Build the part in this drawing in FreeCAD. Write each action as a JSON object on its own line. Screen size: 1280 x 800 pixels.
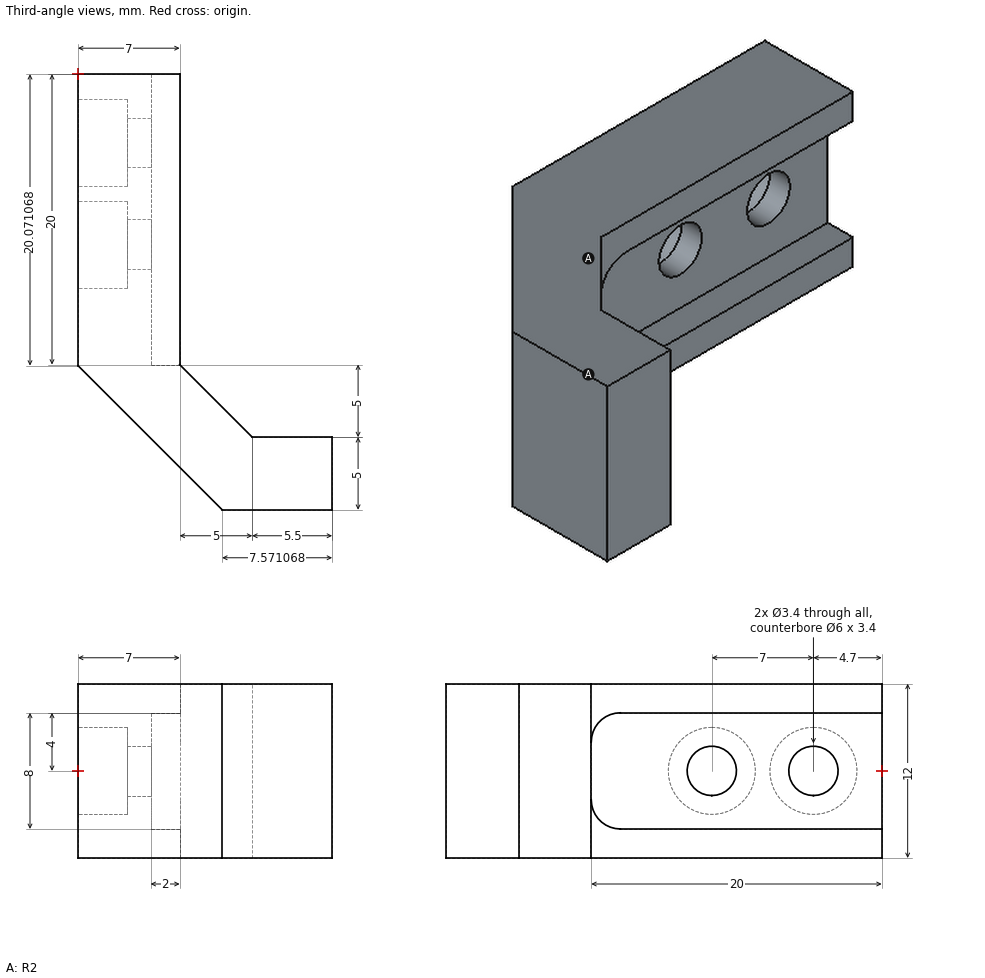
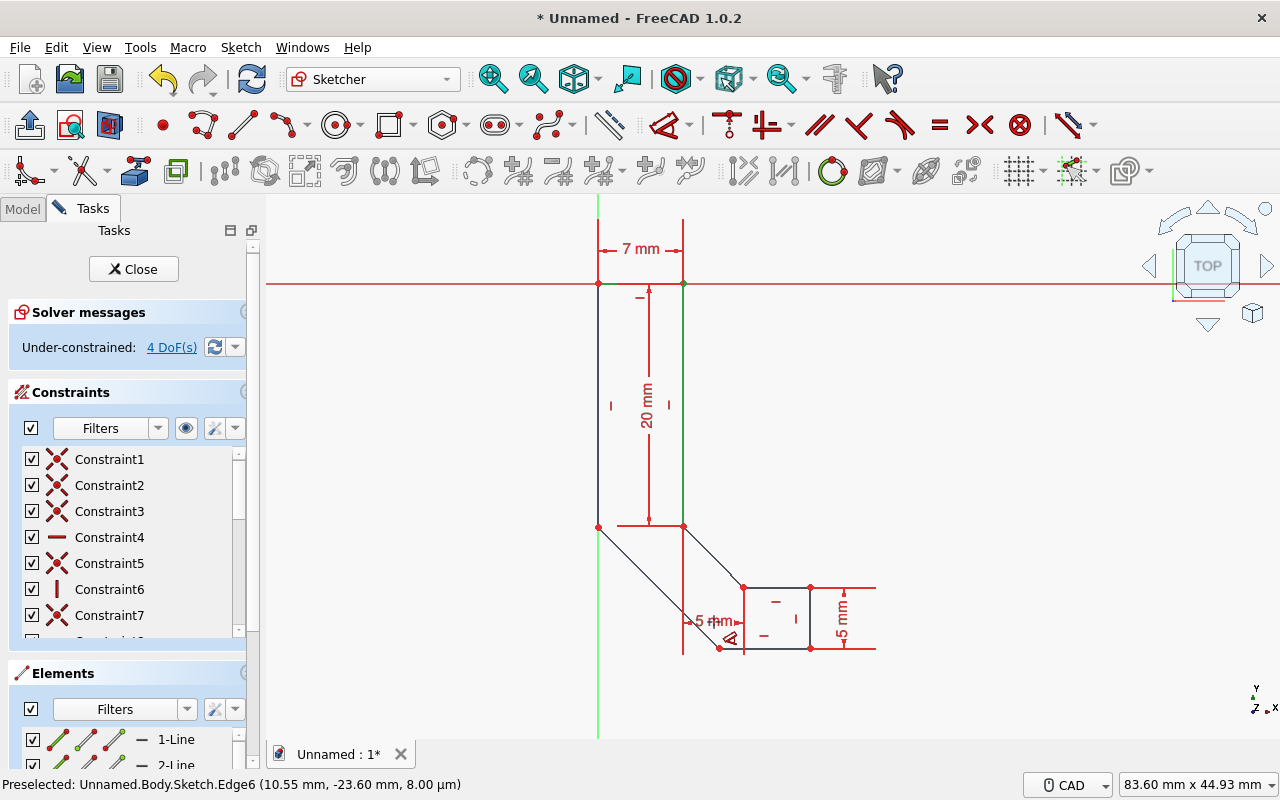
{"action": "left_click", "coordinate": [726, 569]}
{"action": "left_click", "coordinate": [778, 557]}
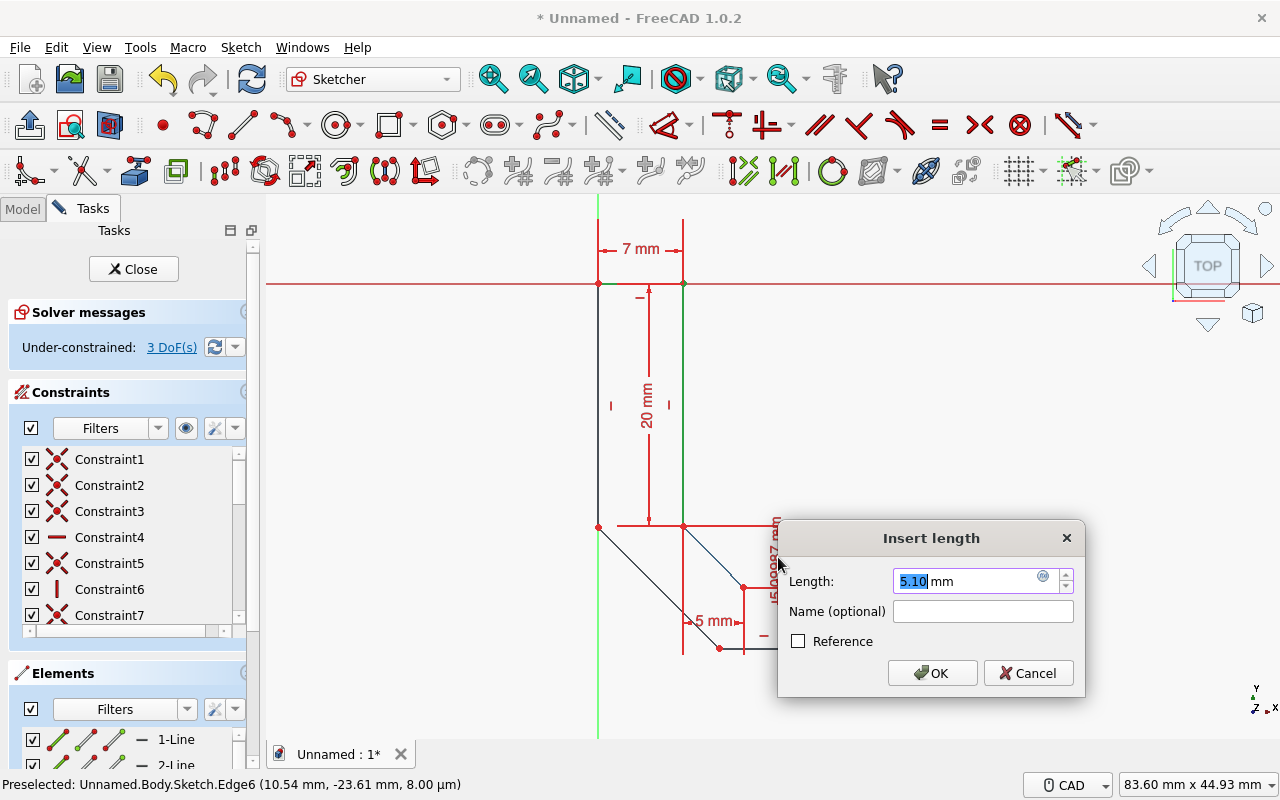
{"action": "type", "text": "5"}
{"action": "key", "text": "Return"}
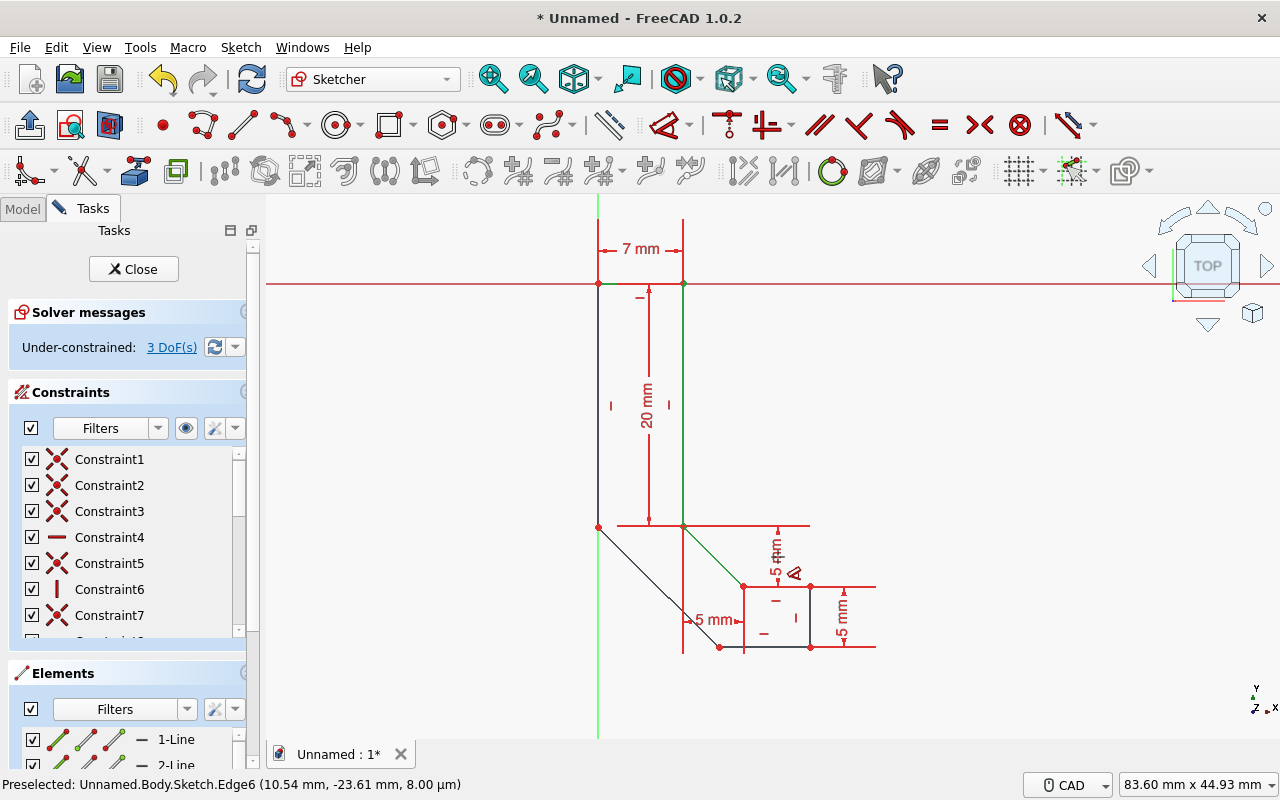
{"action": "left_click", "coordinate": [790, 587]}
{"action": "left_click", "coordinate": [777, 529]}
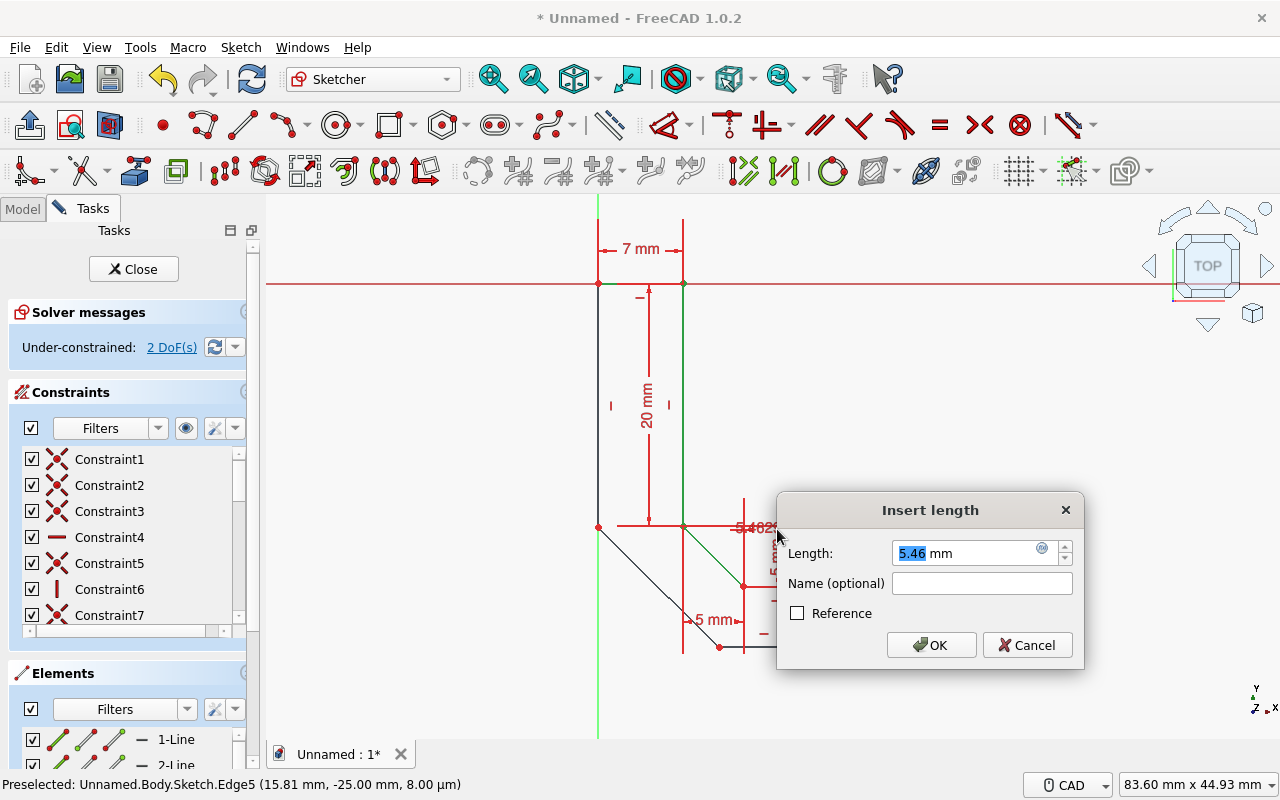
{"action": "type", "text": "5.5"}
{"action": "key", "text": "Return"}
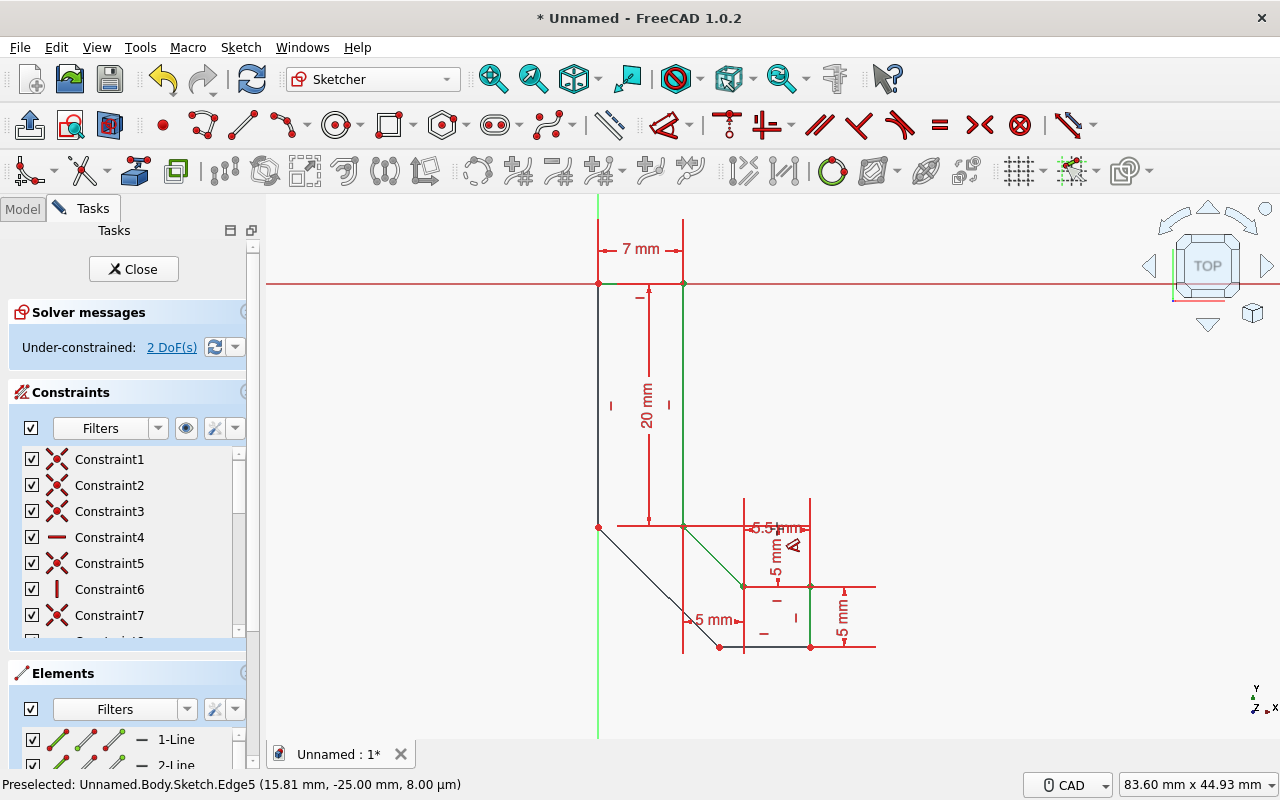
{"action": "left_click", "coordinate": [746, 647]}
{"action": "left_click", "coordinate": [765, 681]}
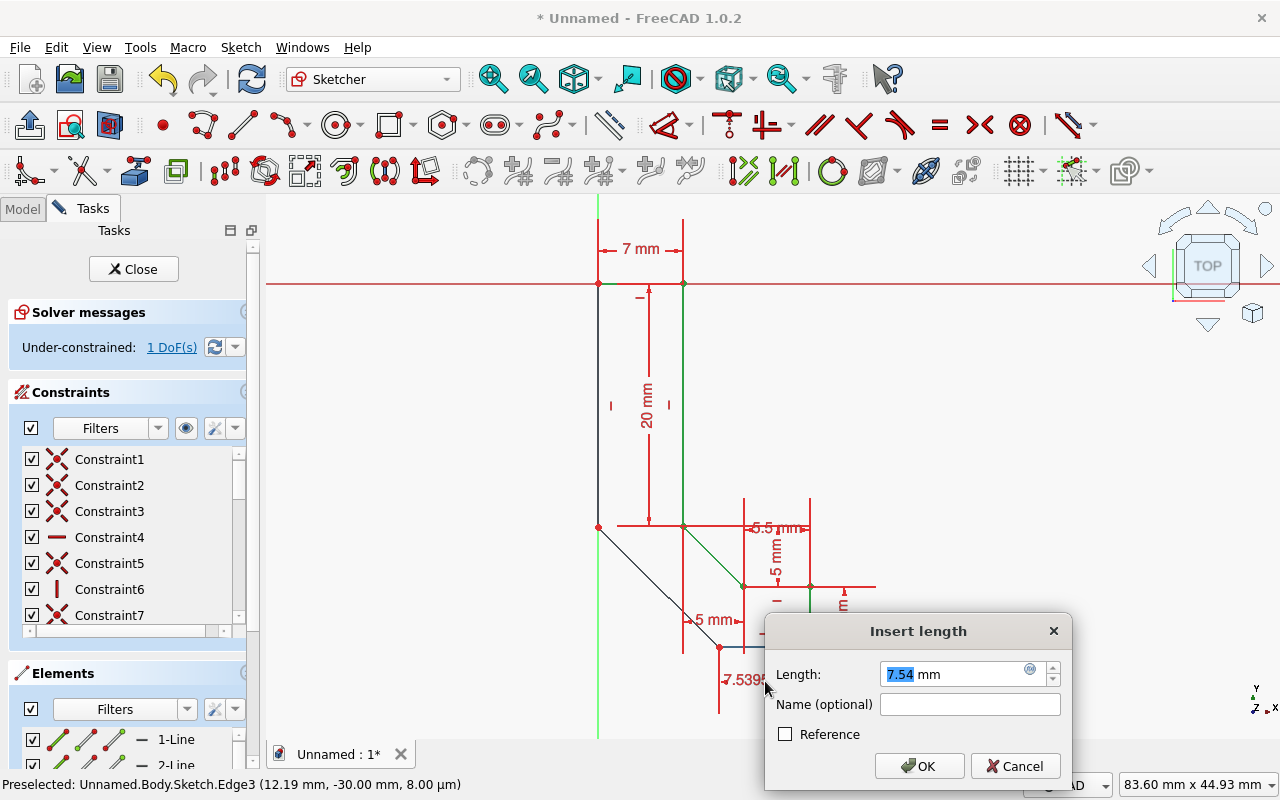
{"action": "type", "text": "7.571068"}
{"action": "key", "text": "Return"}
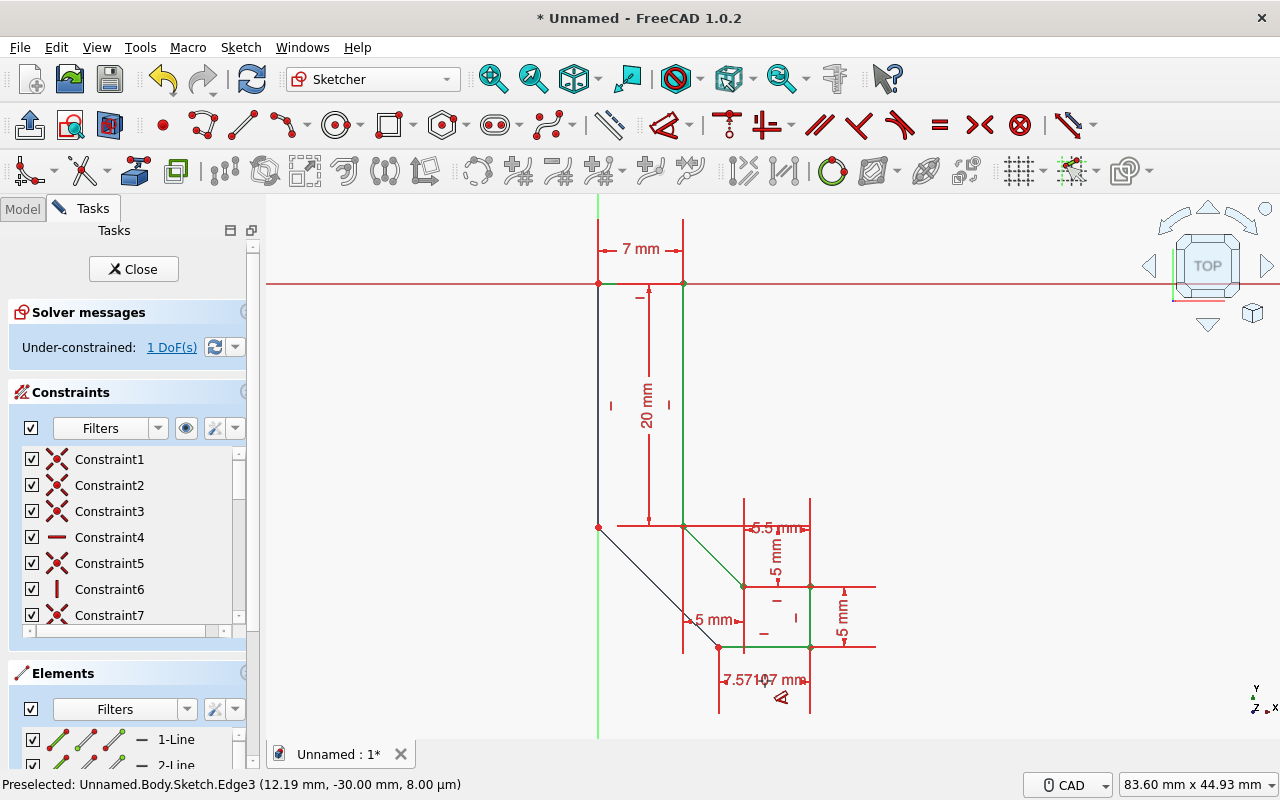
{"action": "left_click", "coordinate": [598, 357]}
{"action": "left_click", "coordinate": [564, 406]}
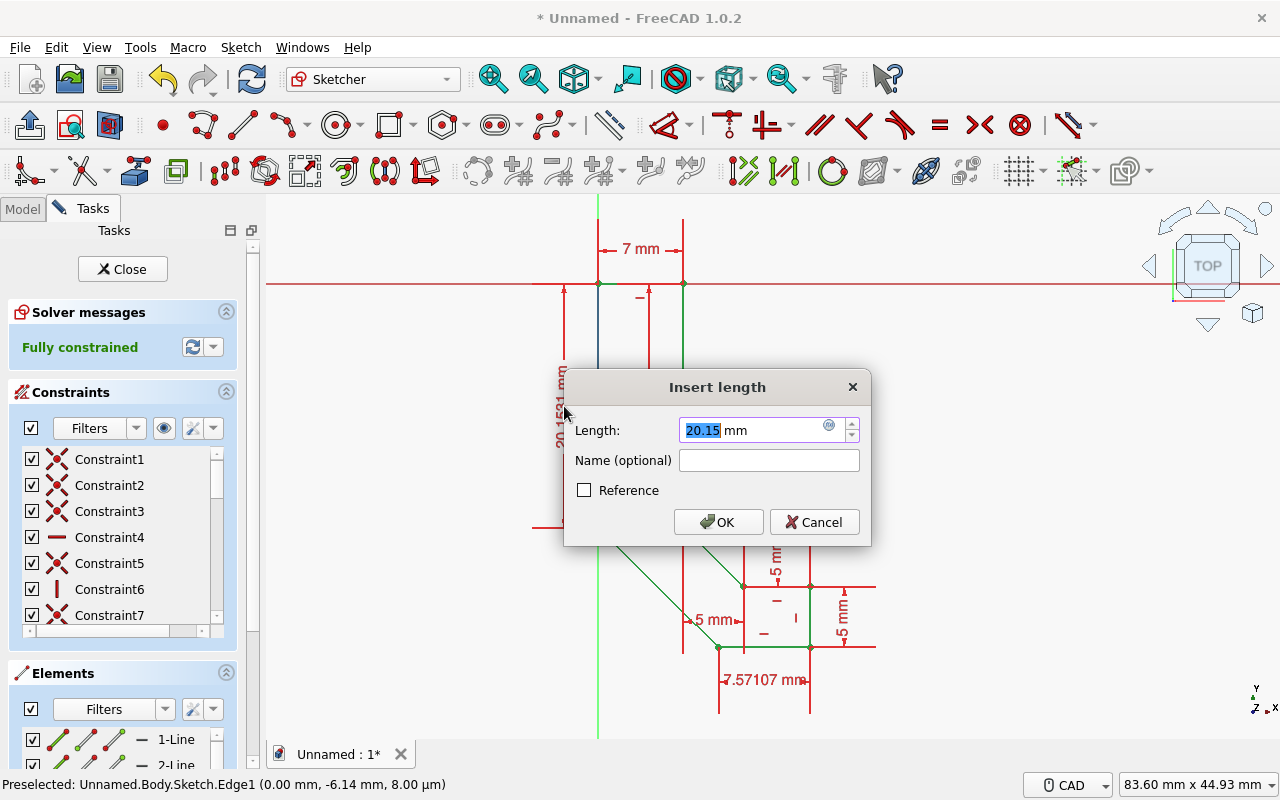
{"action": "type", "text": "20.071068"}
{"action": "key", "text": "Return"}
{"action": "key", "text": "Escape"}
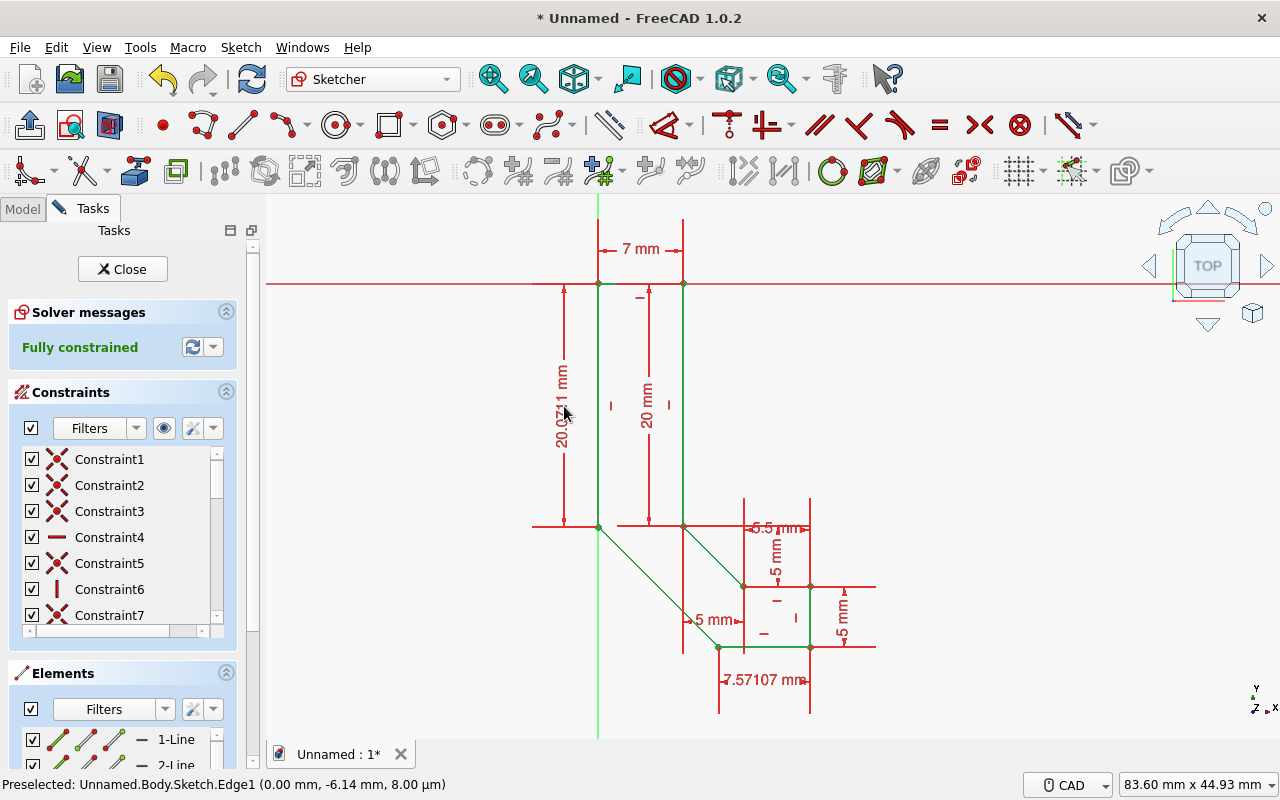
{"action": "left_click", "coordinate": [123, 269]}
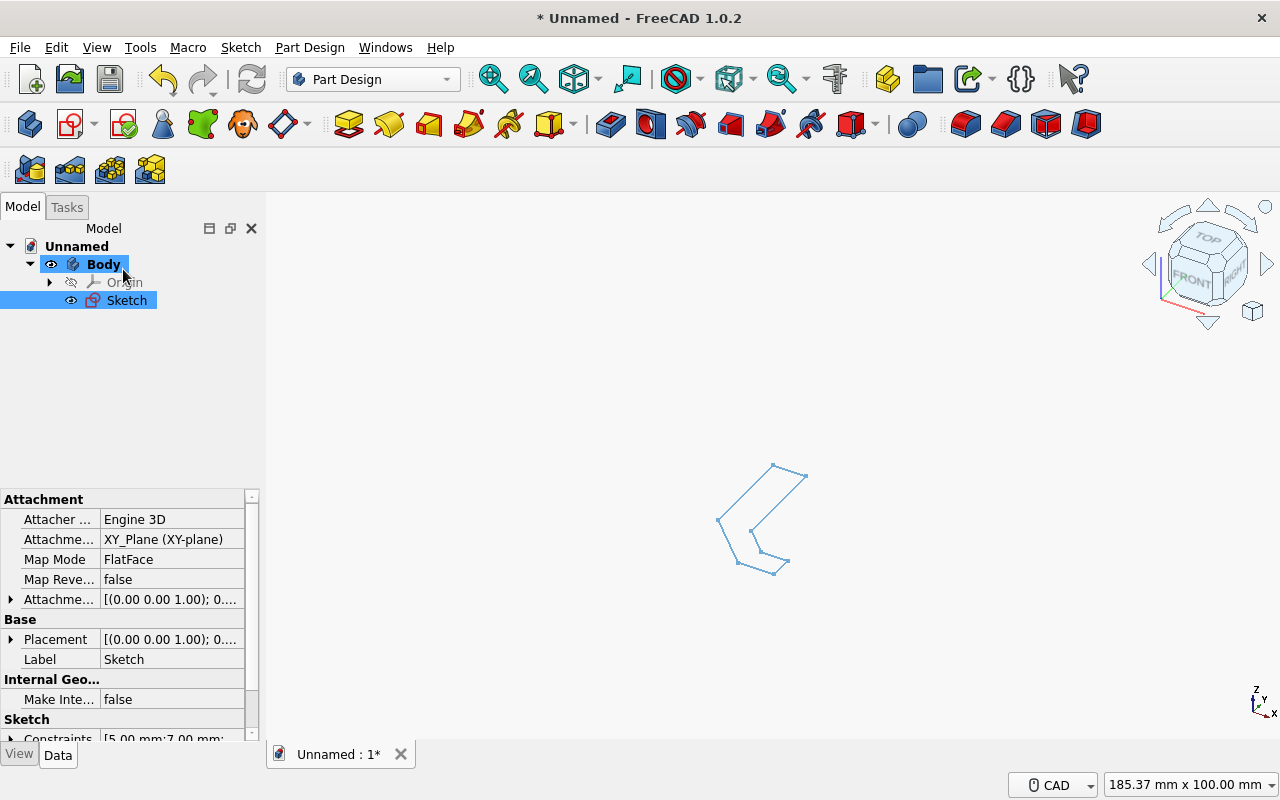
{"action": "left_click", "coordinate": [350, 124]}